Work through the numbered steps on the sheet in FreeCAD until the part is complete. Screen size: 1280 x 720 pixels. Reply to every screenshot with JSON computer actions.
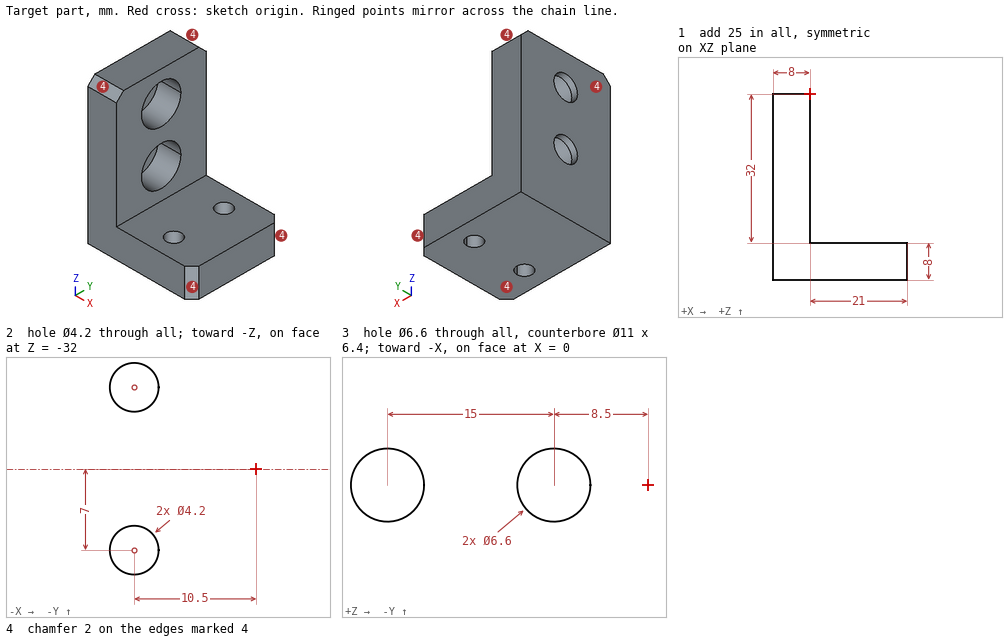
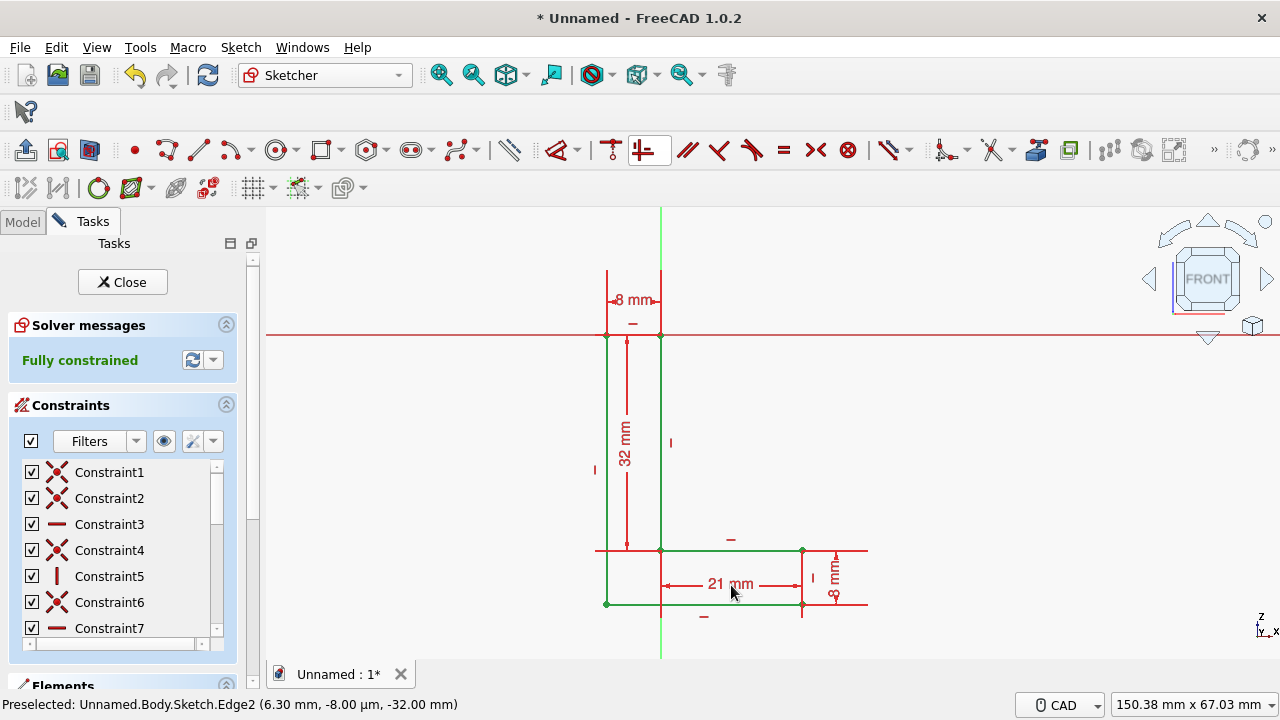
{"action": "left_click", "coordinate": [123, 282]}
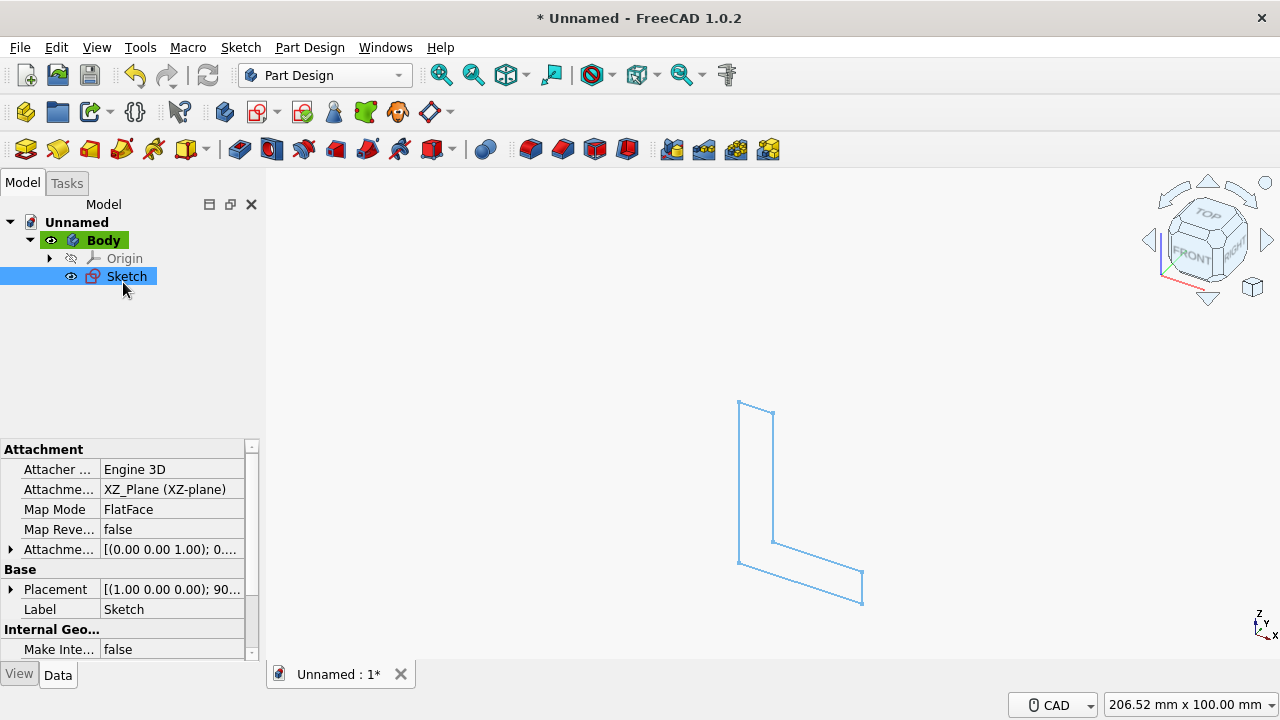
{"action": "left_click", "coordinate": [26, 150]}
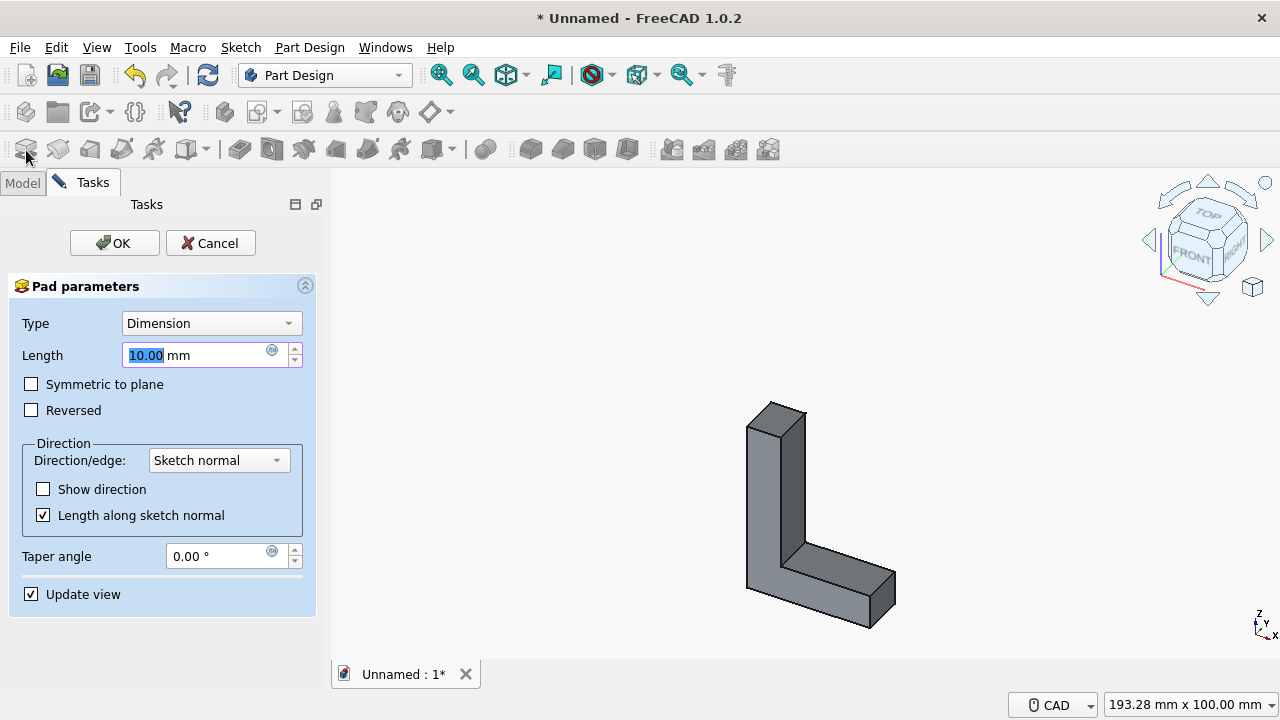
{"action": "type", "text": "25"}
{"action": "key", "text": "Tab"}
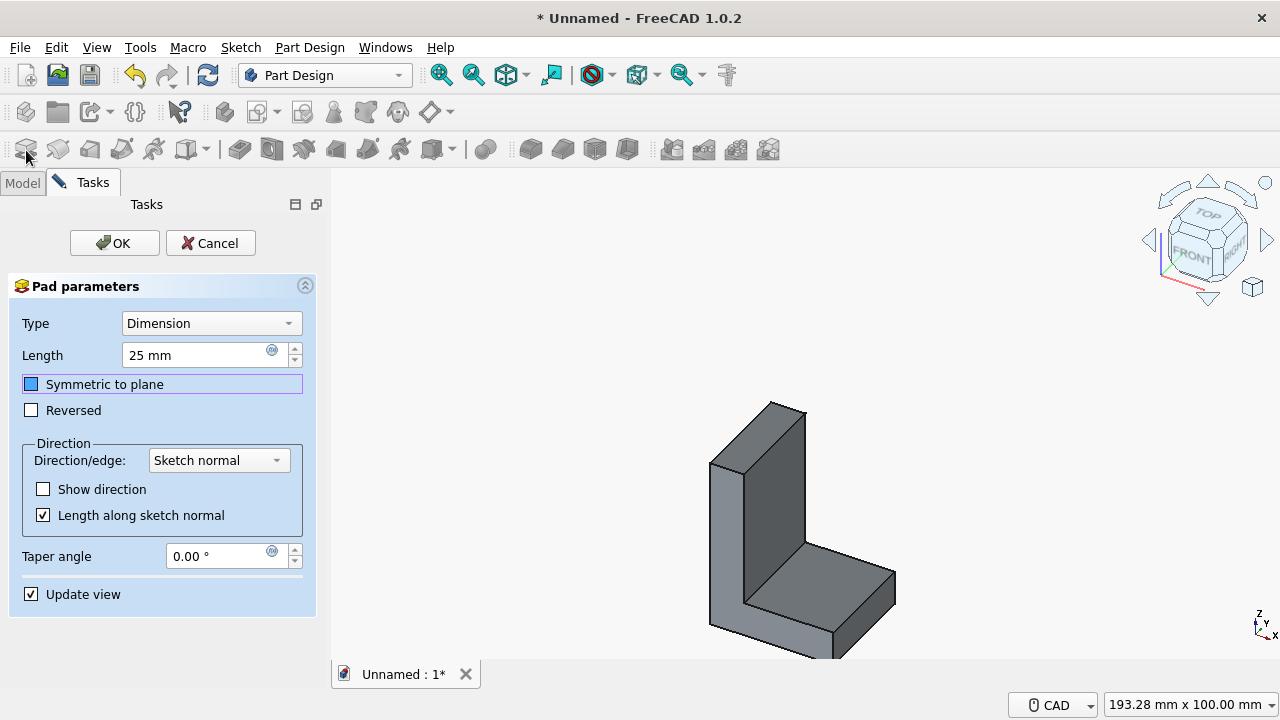
{"action": "left_click", "coordinate": [30, 384]}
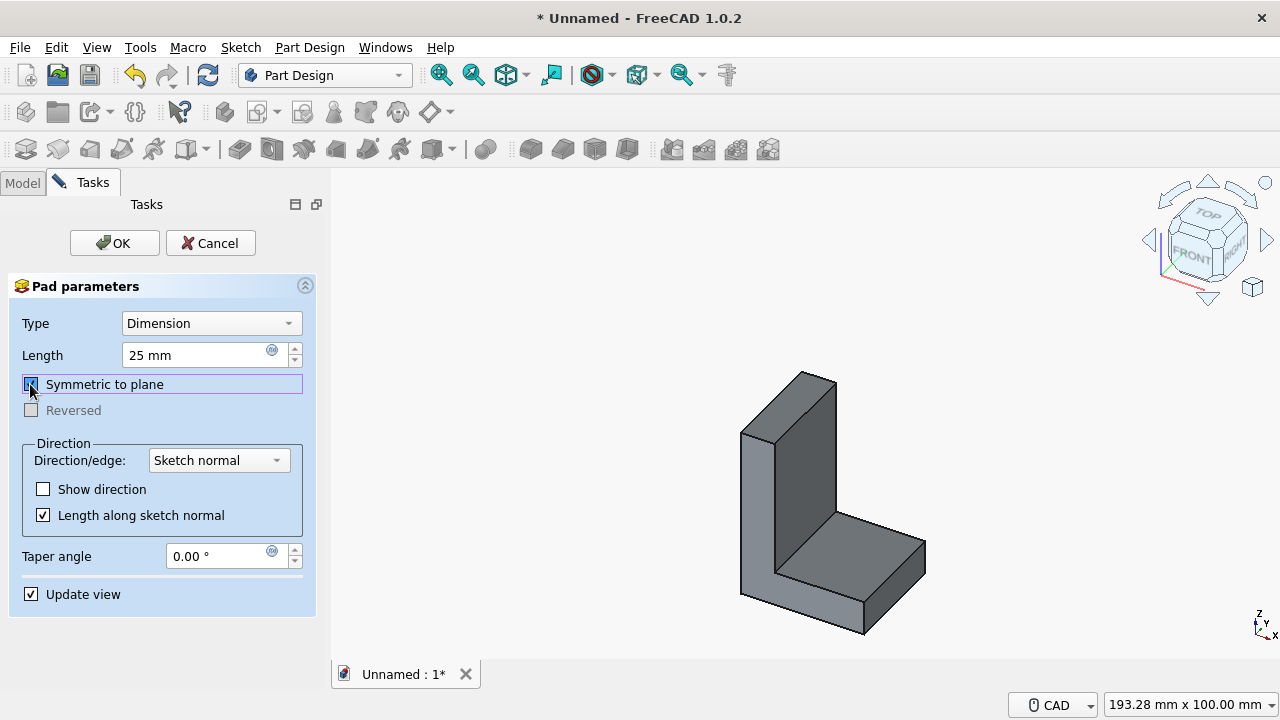
{"action": "left_click", "coordinate": [115, 243]}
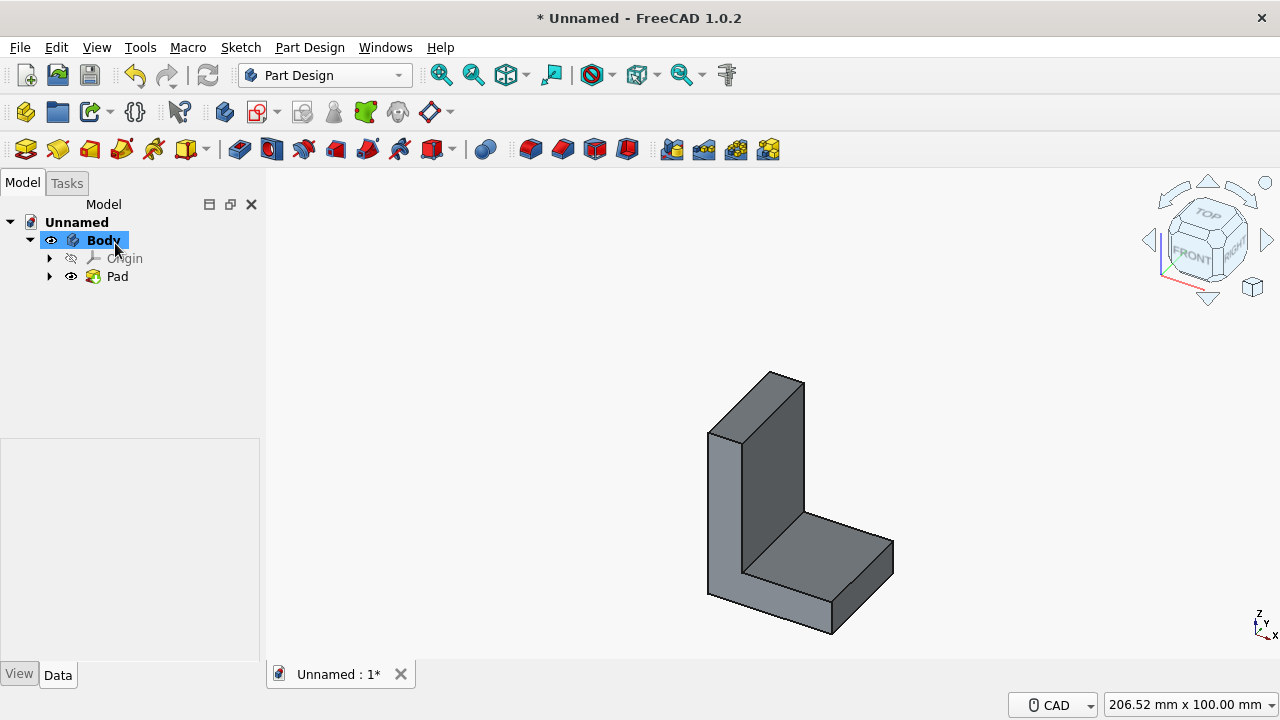
{"action": "left_click", "coordinate": [818, 556]}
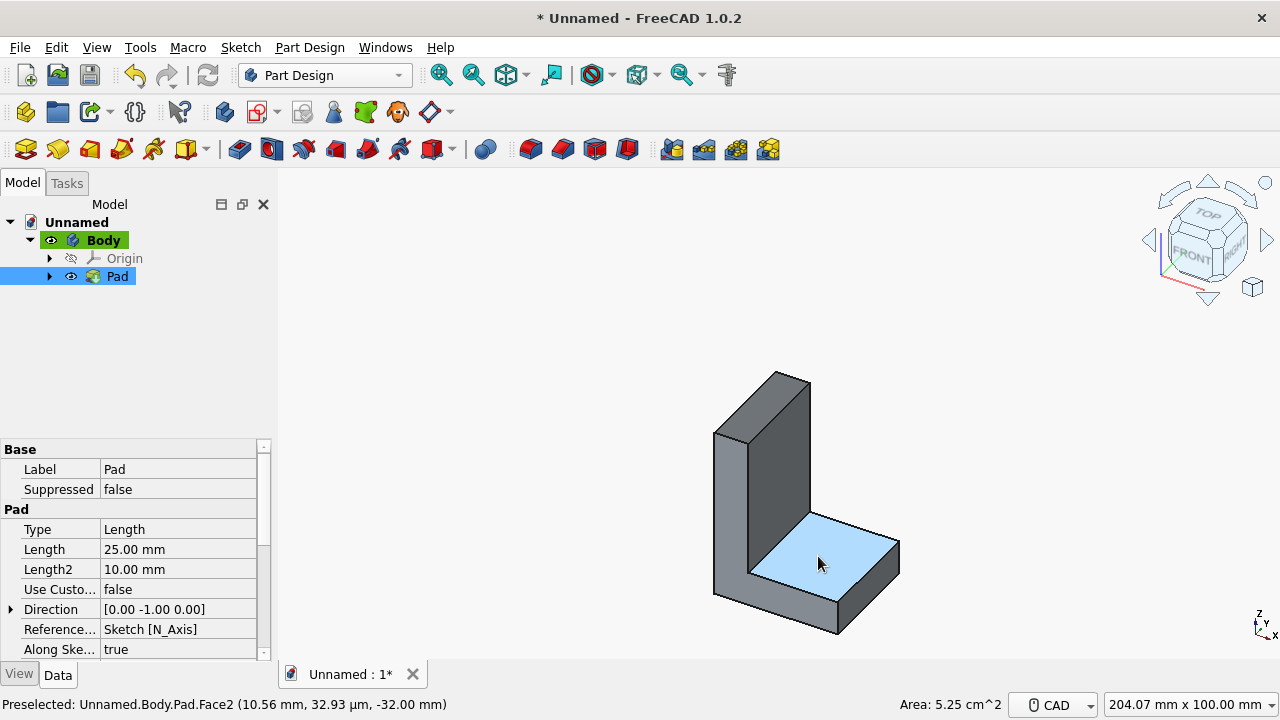
{"action": "left_click", "coordinate": [258, 112]}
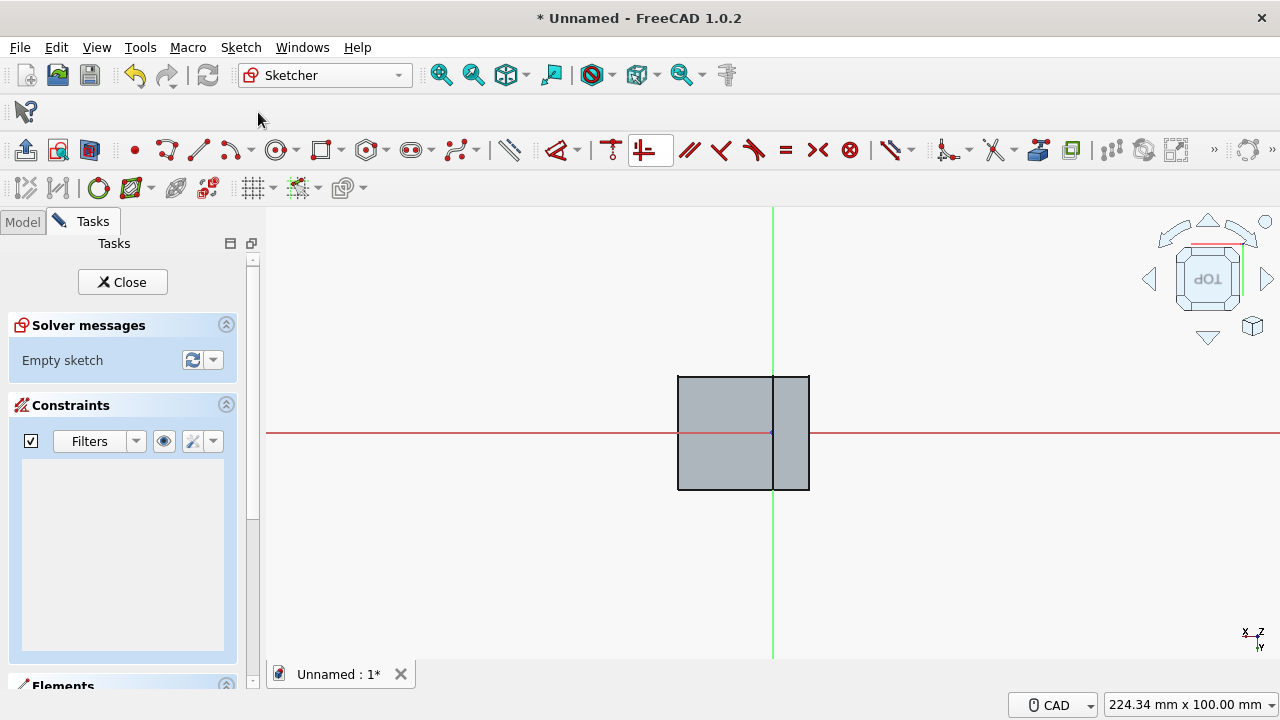
{"action": "scroll", "coordinate": [762, 433], "scroll_direction": "up", "scroll_amount": 6}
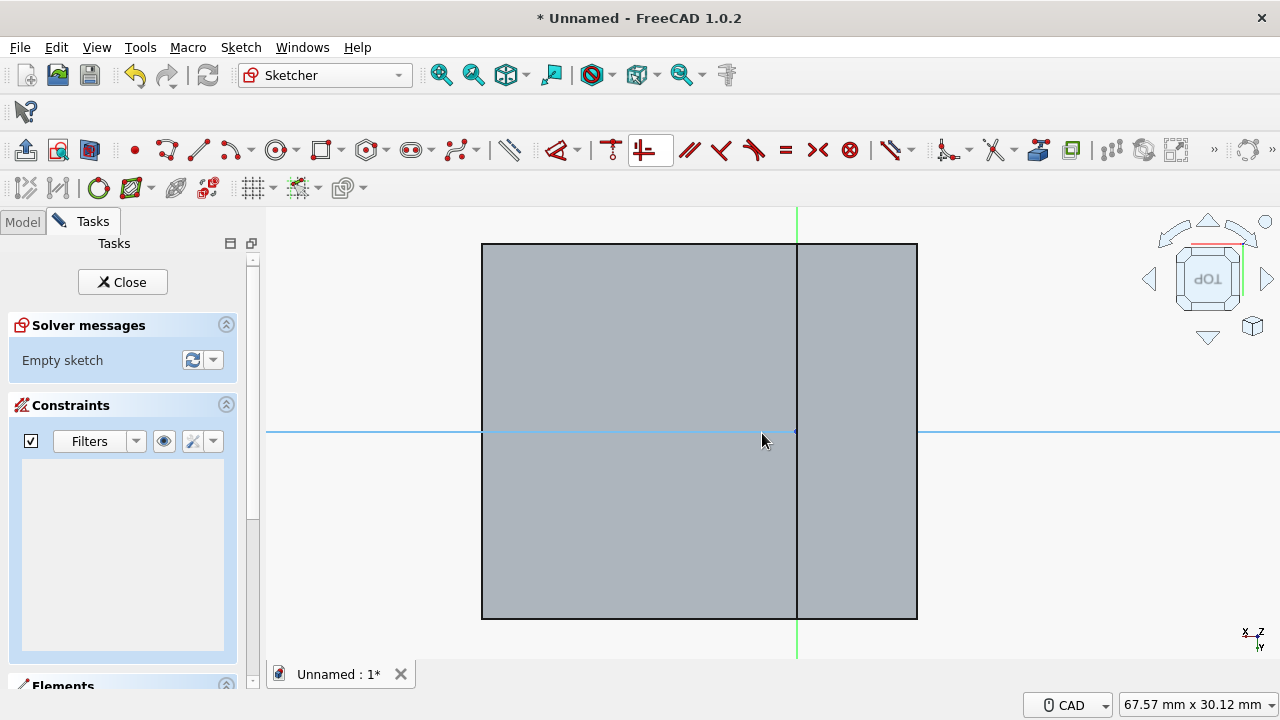
{"action": "left_click", "coordinate": [276, 150]}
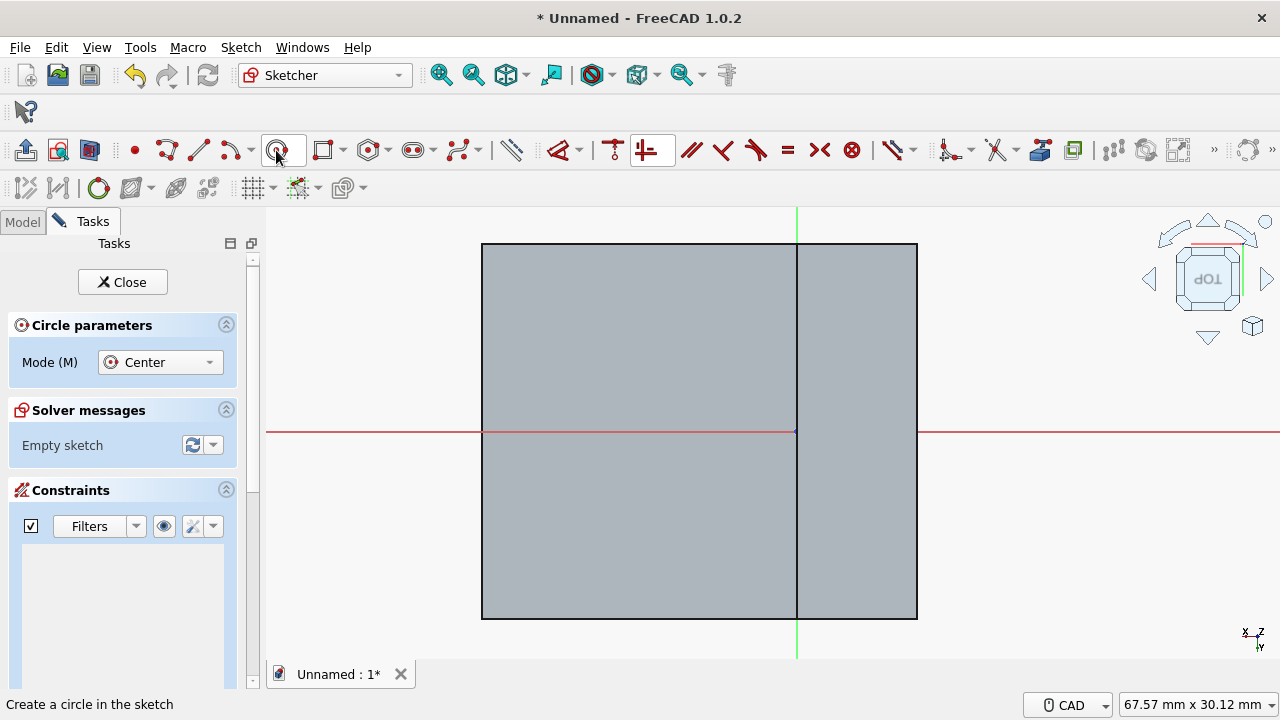
{"action": "left_click", "coordinate": [640, 537]}
{"action": "left_click", "coordinate": [662, 515]}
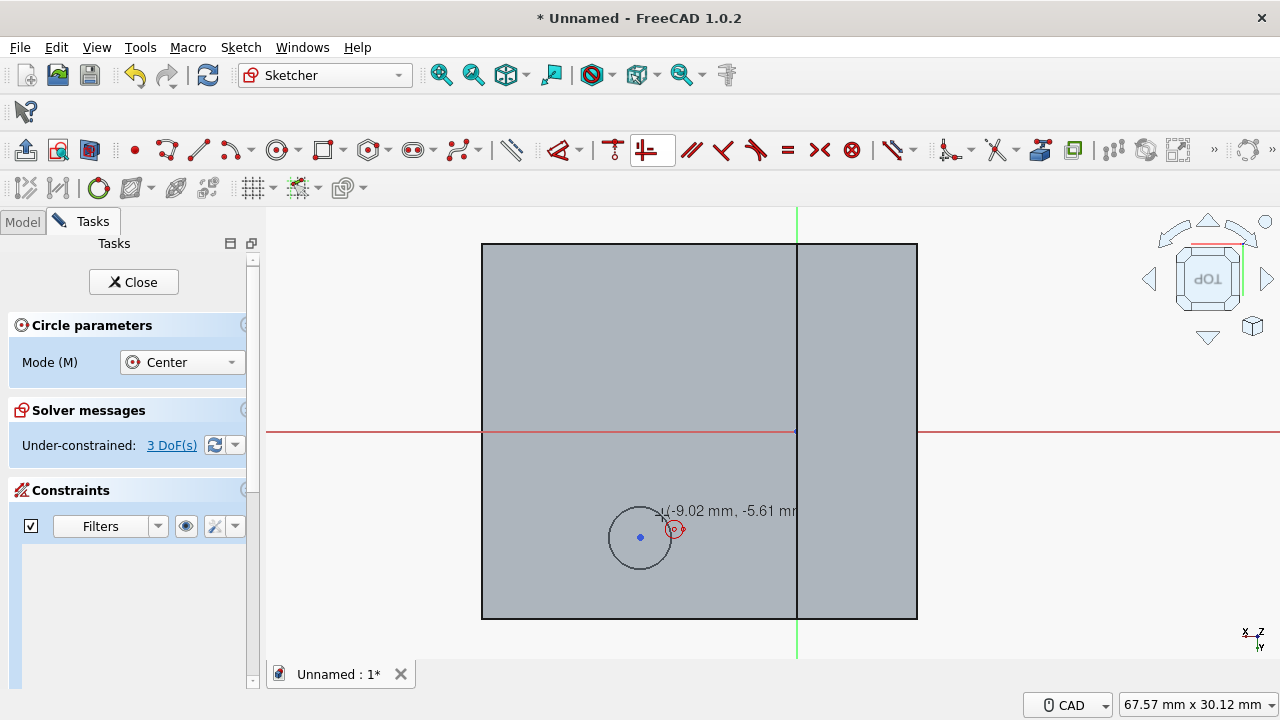
{"action": "left_click", "coordinate": [640, 327]}
{"action": "left_click", "coordinate": [662, 305]}
{"action": "key", "text": "Escape"}